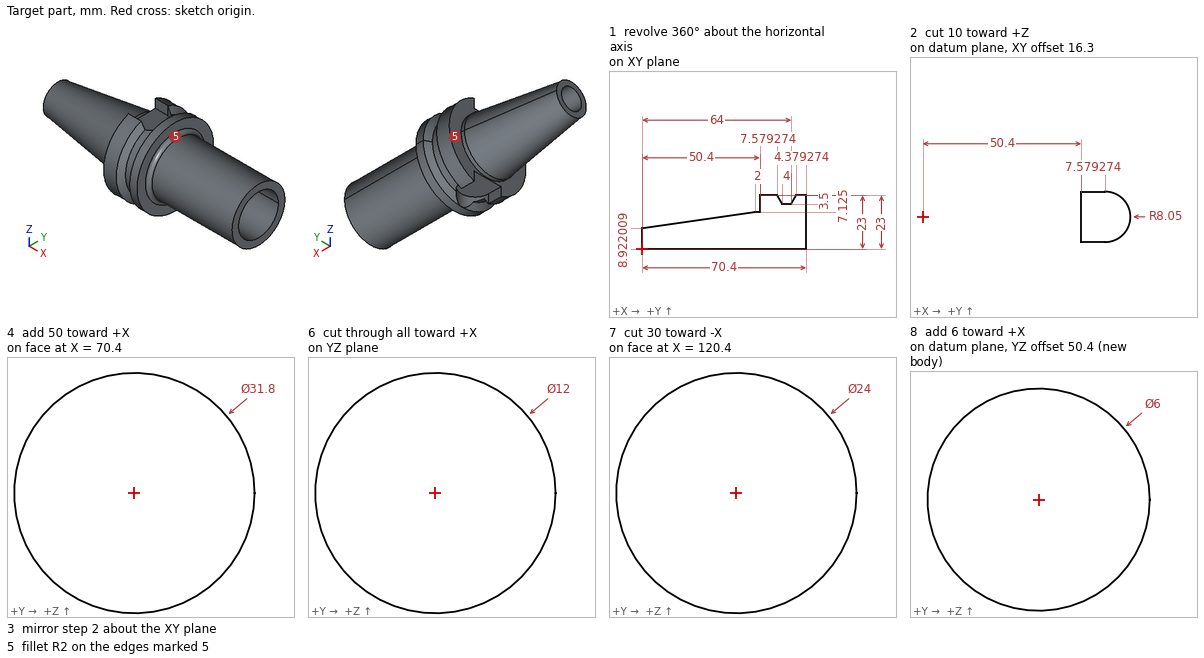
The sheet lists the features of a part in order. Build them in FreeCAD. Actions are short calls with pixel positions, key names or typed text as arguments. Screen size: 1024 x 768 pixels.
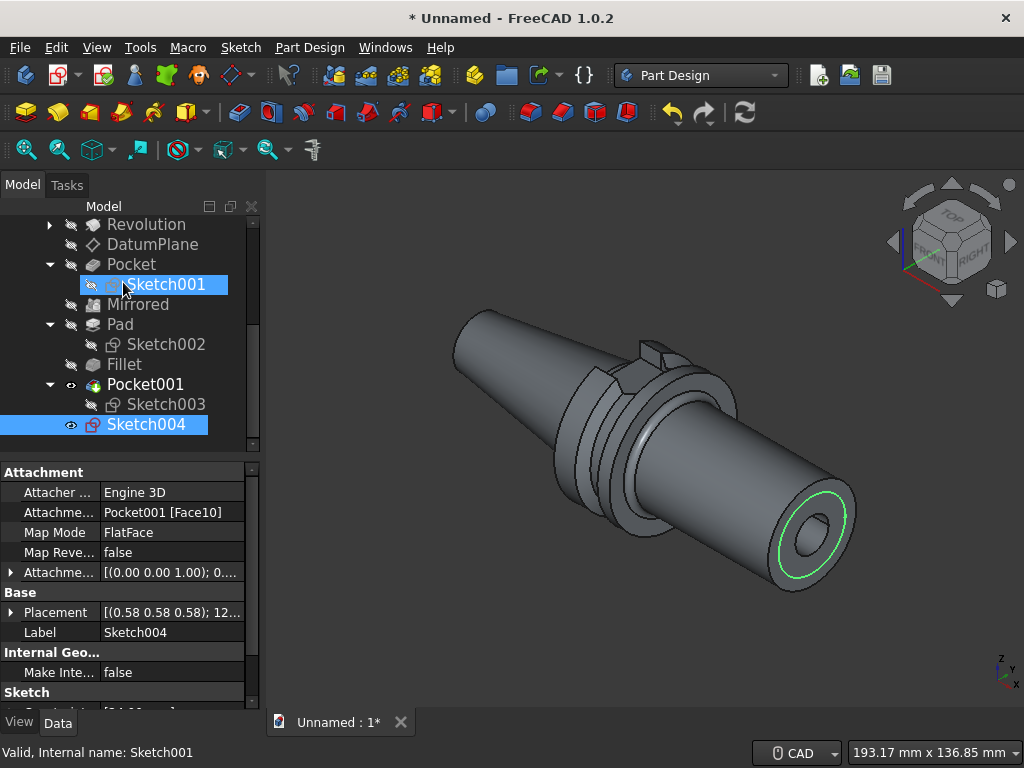
click(240, 112)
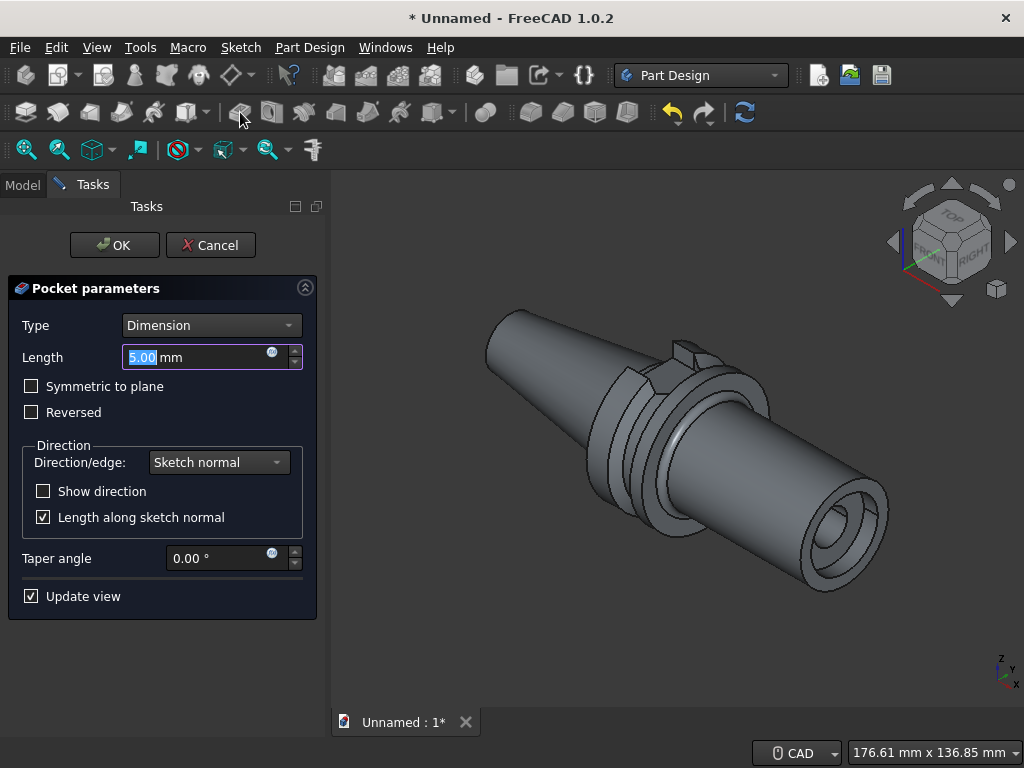
text(30)
key(Tab)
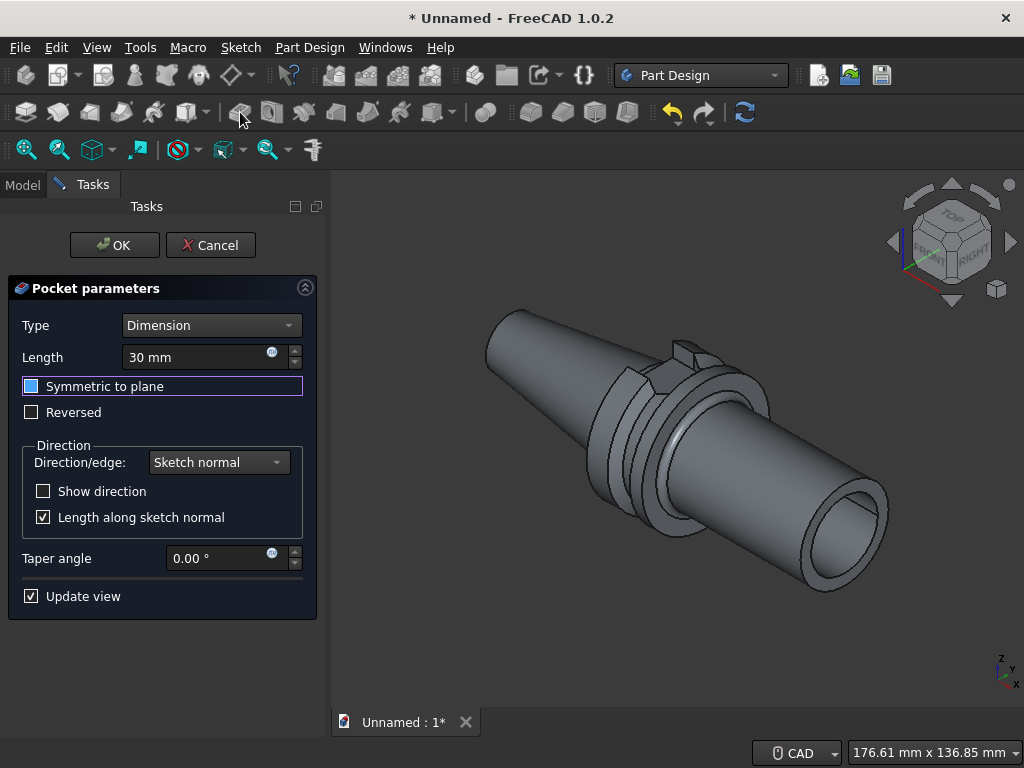
click(115, 245)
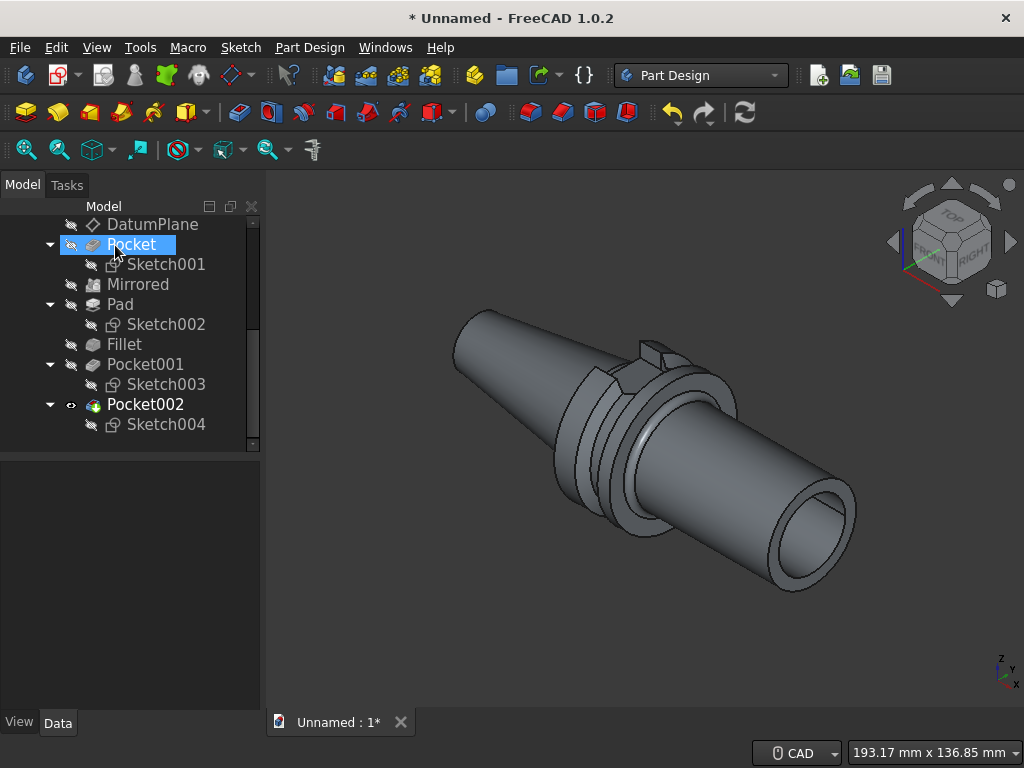
click(26, 76)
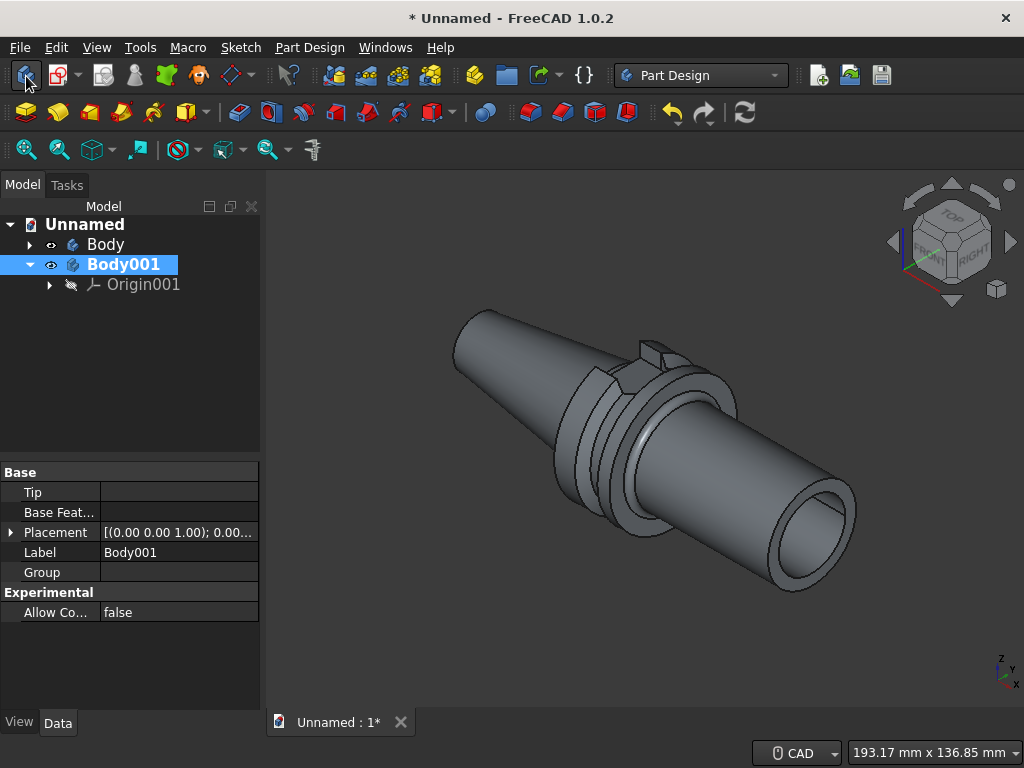
click(50, 285)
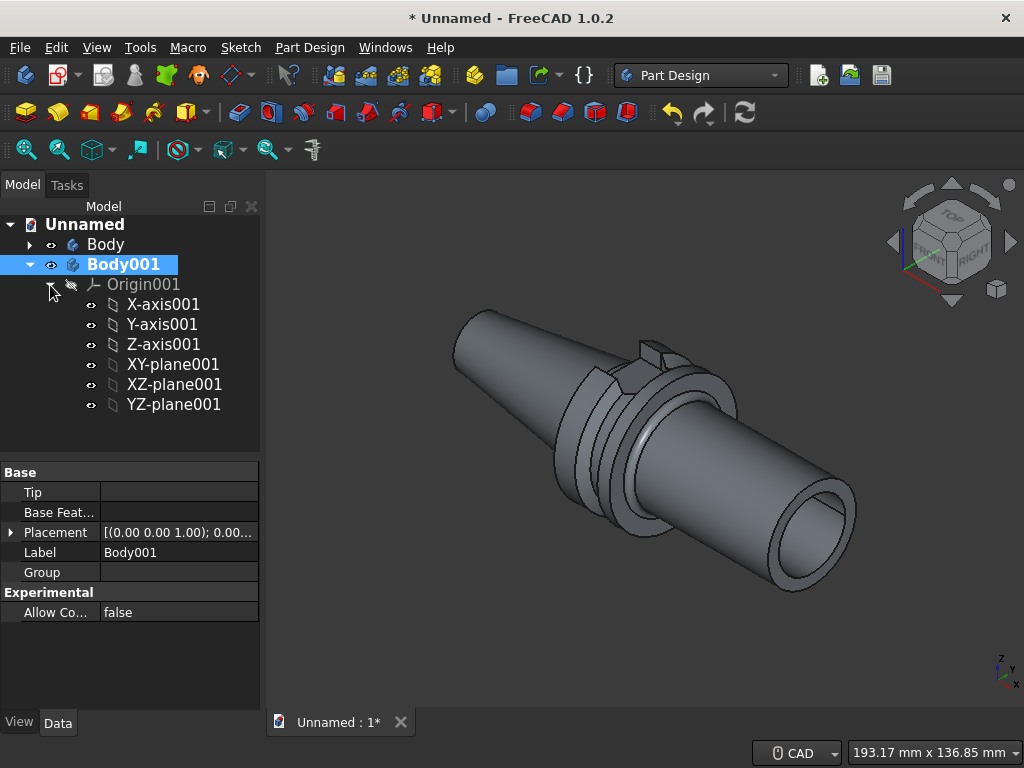
click(136, 405)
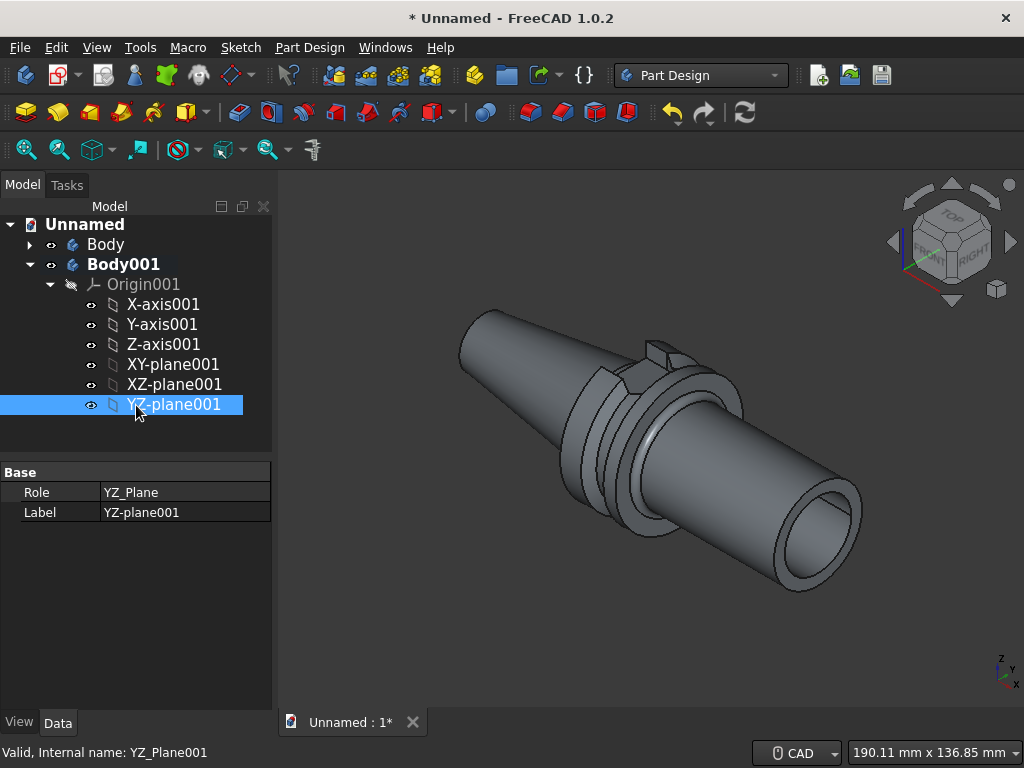
click(232, 76)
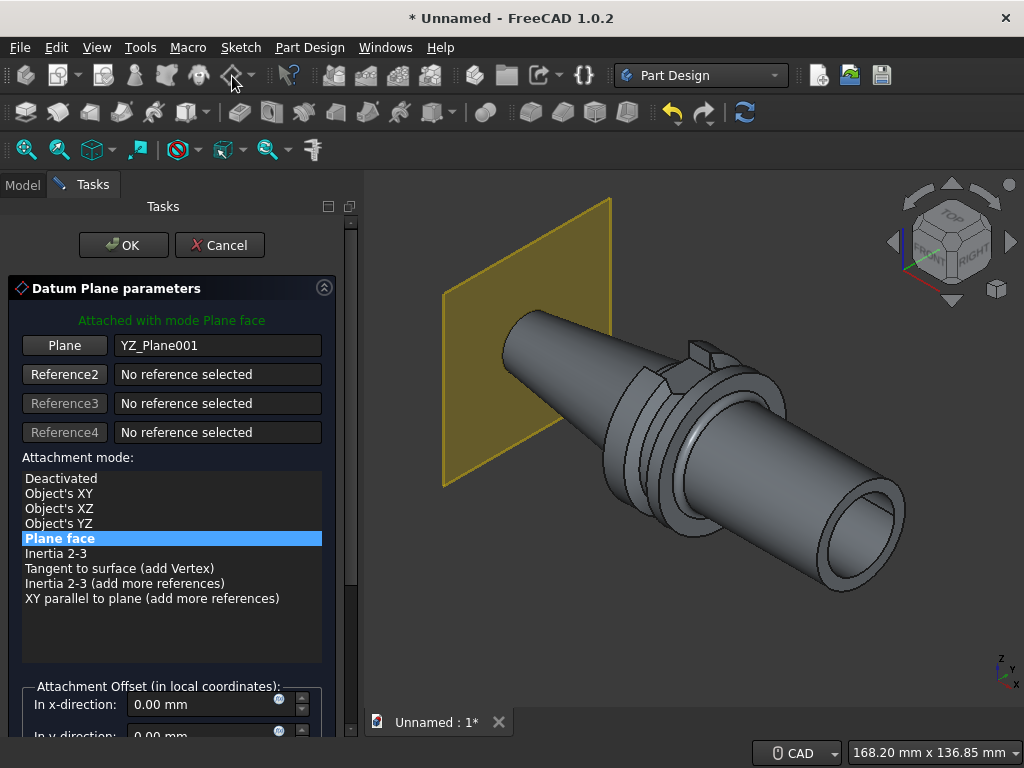
scroll(351, 476, down, 2)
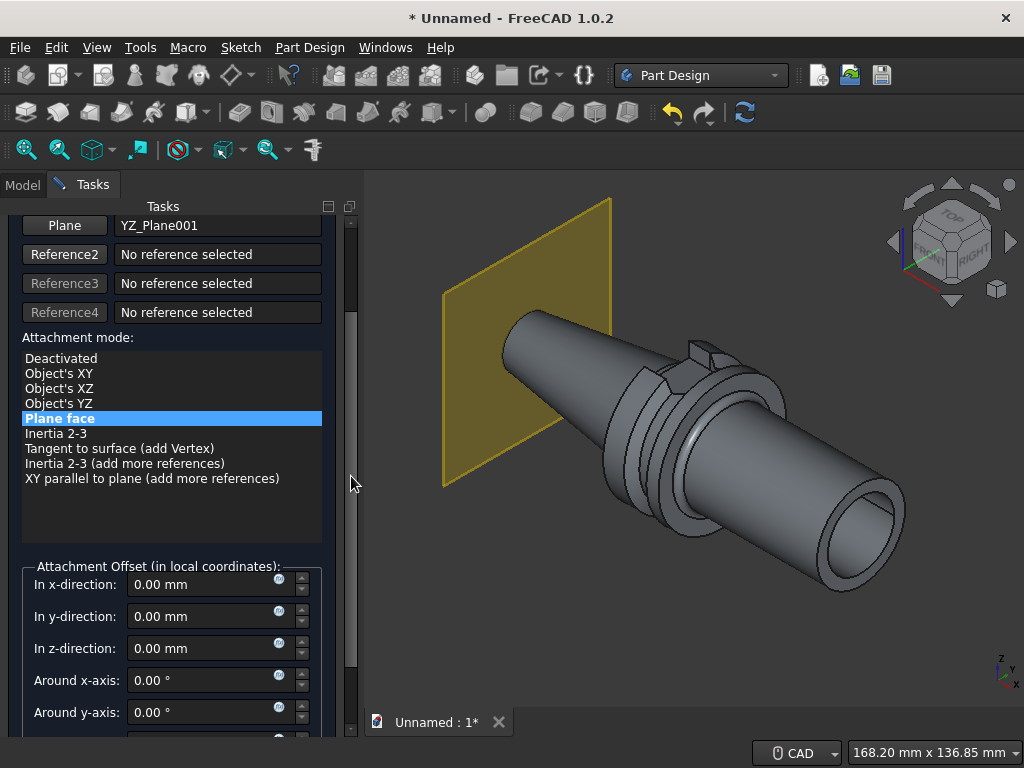
triple_click(210, 648)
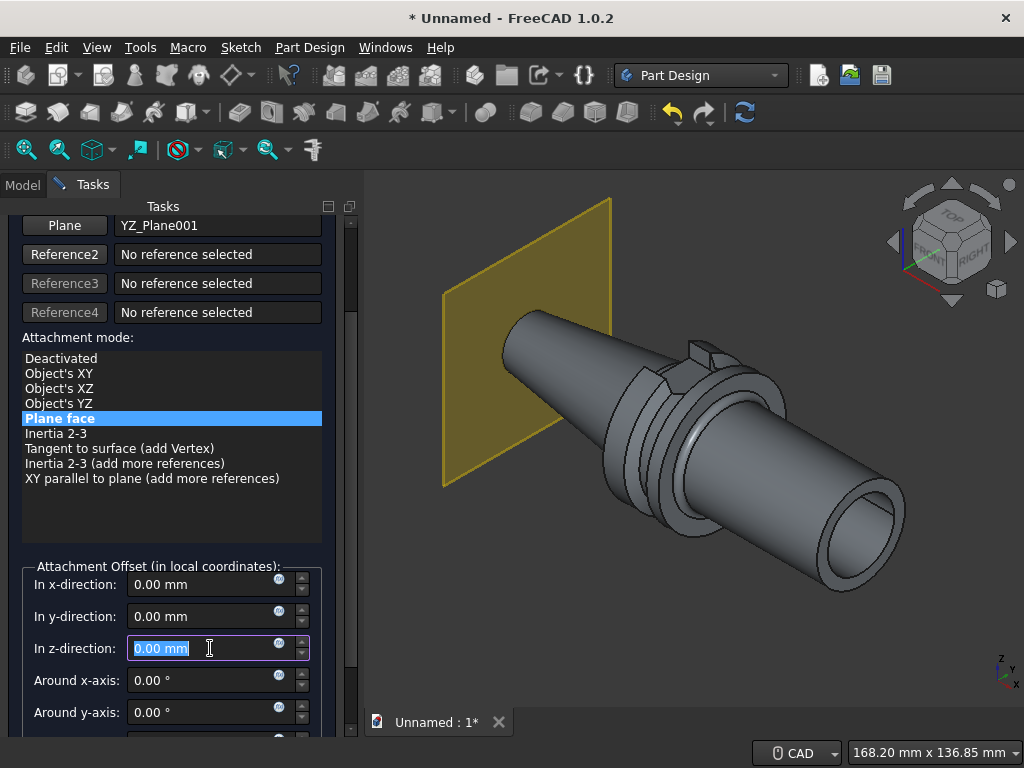
text(50.4)
key(Tab)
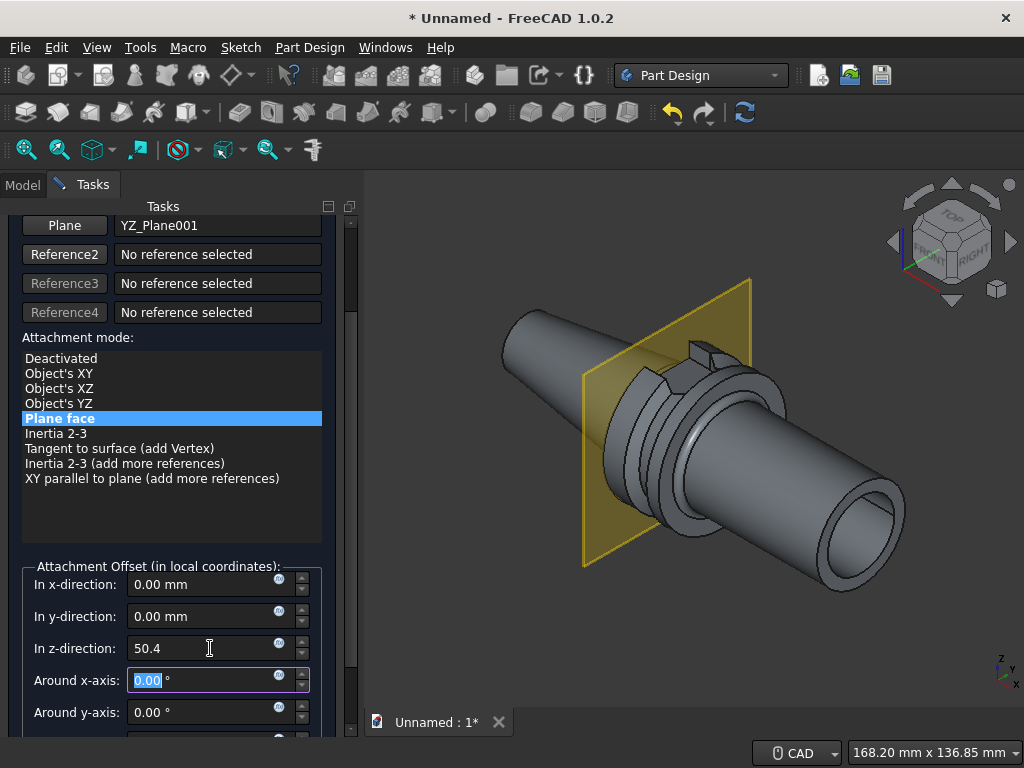
scroll(351, 476, up, 3)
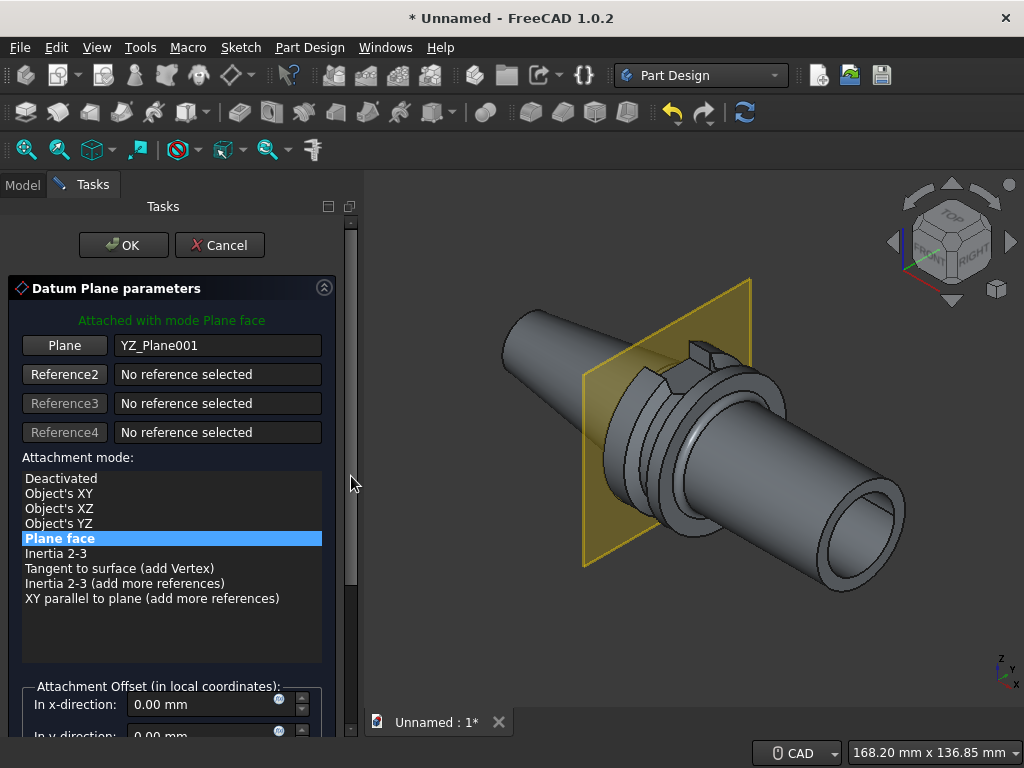
click(124, 245)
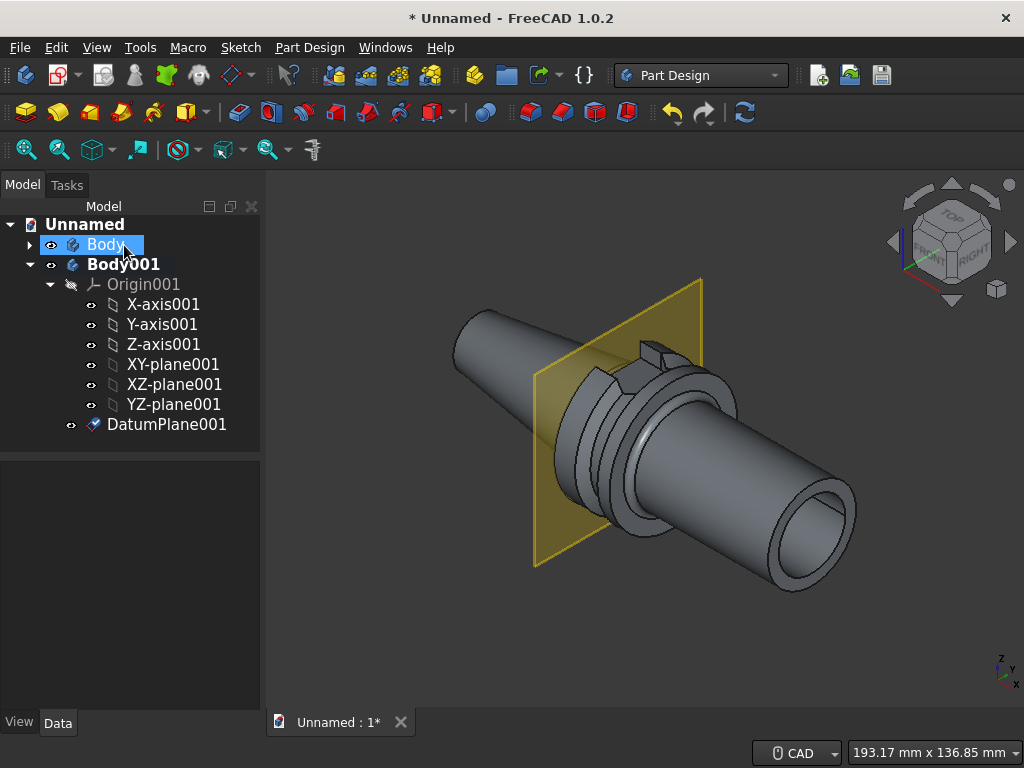
click(116, 425)